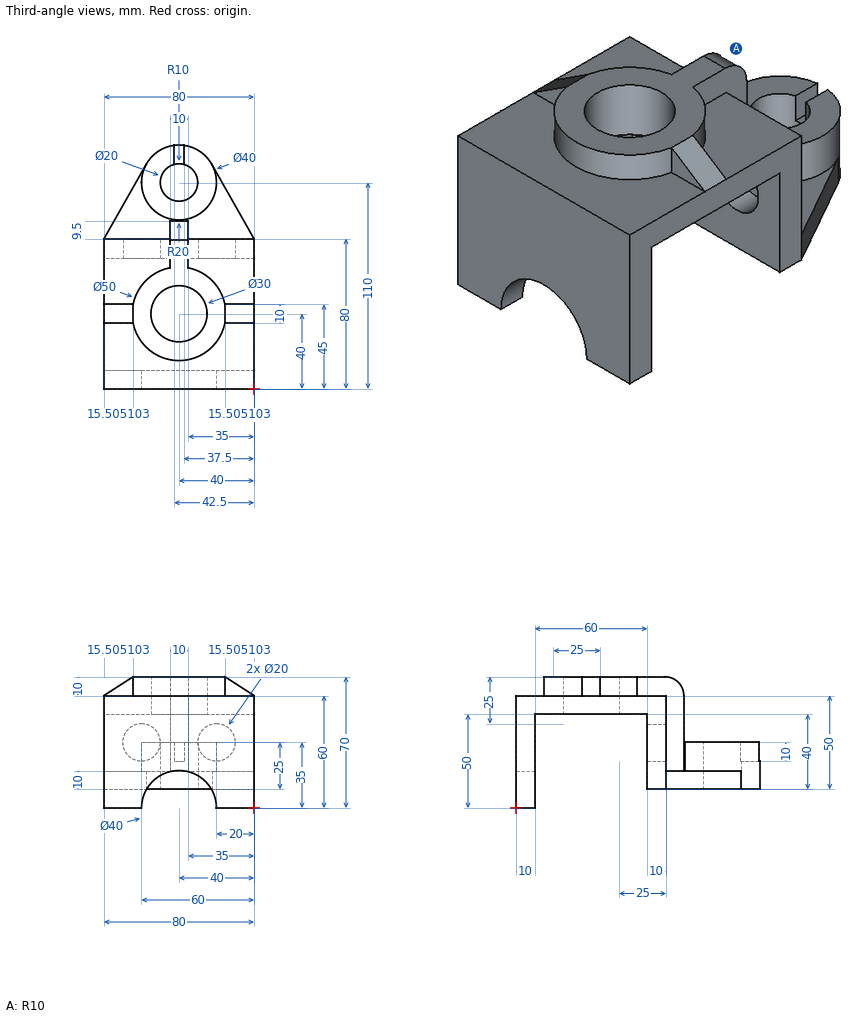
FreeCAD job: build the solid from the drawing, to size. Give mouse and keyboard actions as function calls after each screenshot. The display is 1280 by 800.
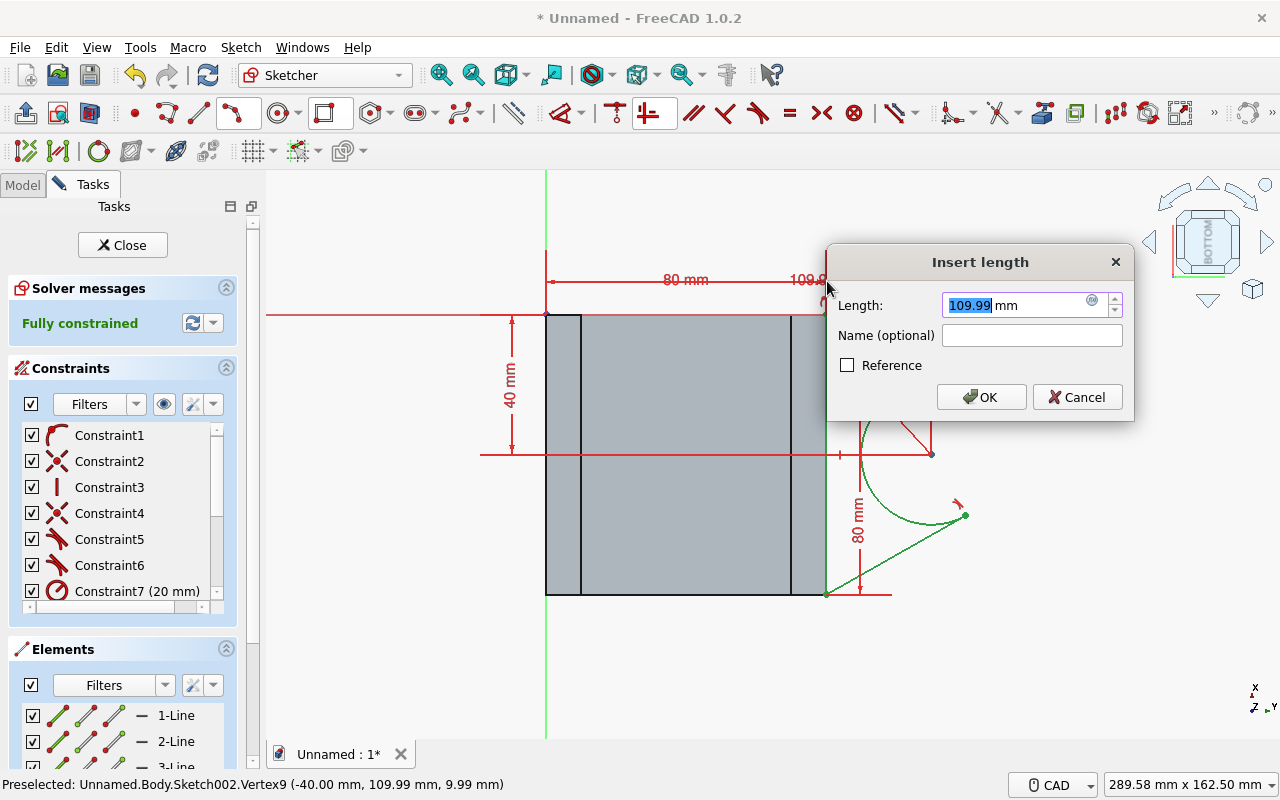
text(110)
key(Return)
key(Escape)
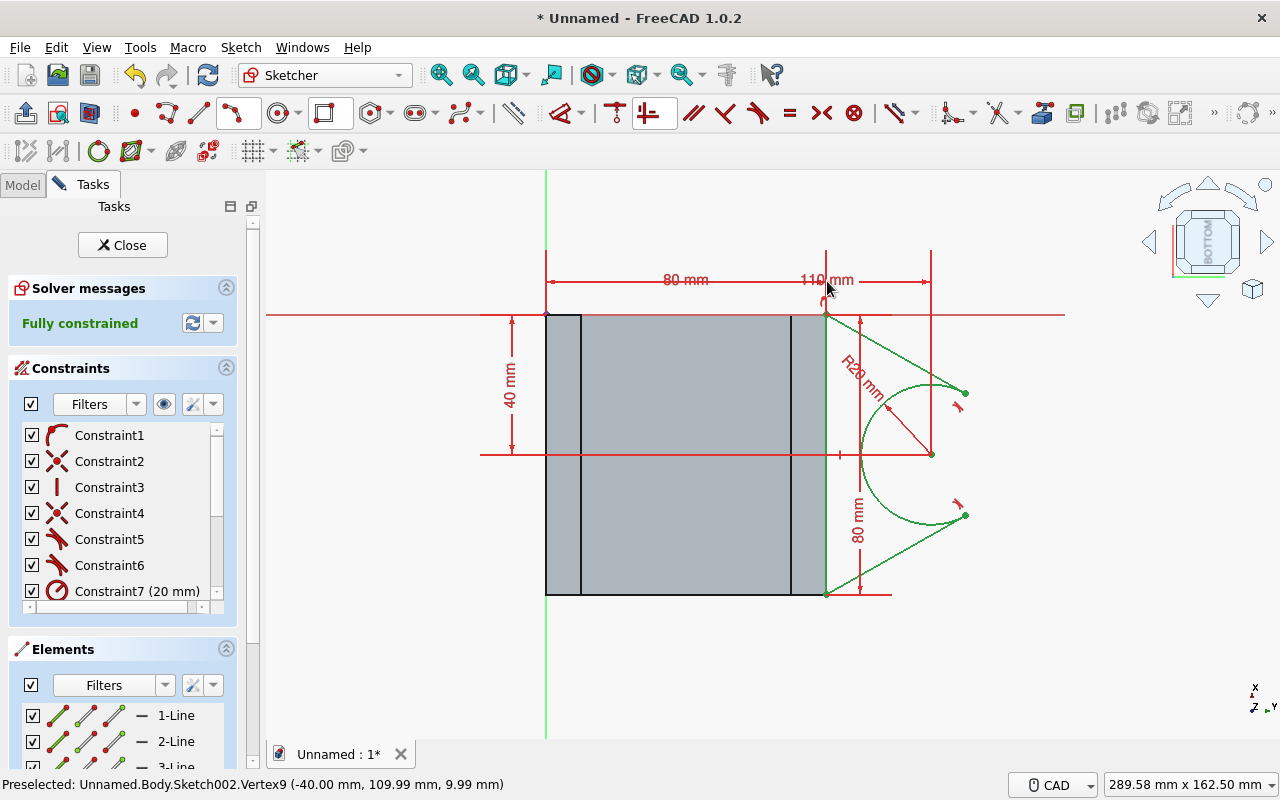
click(123, 245)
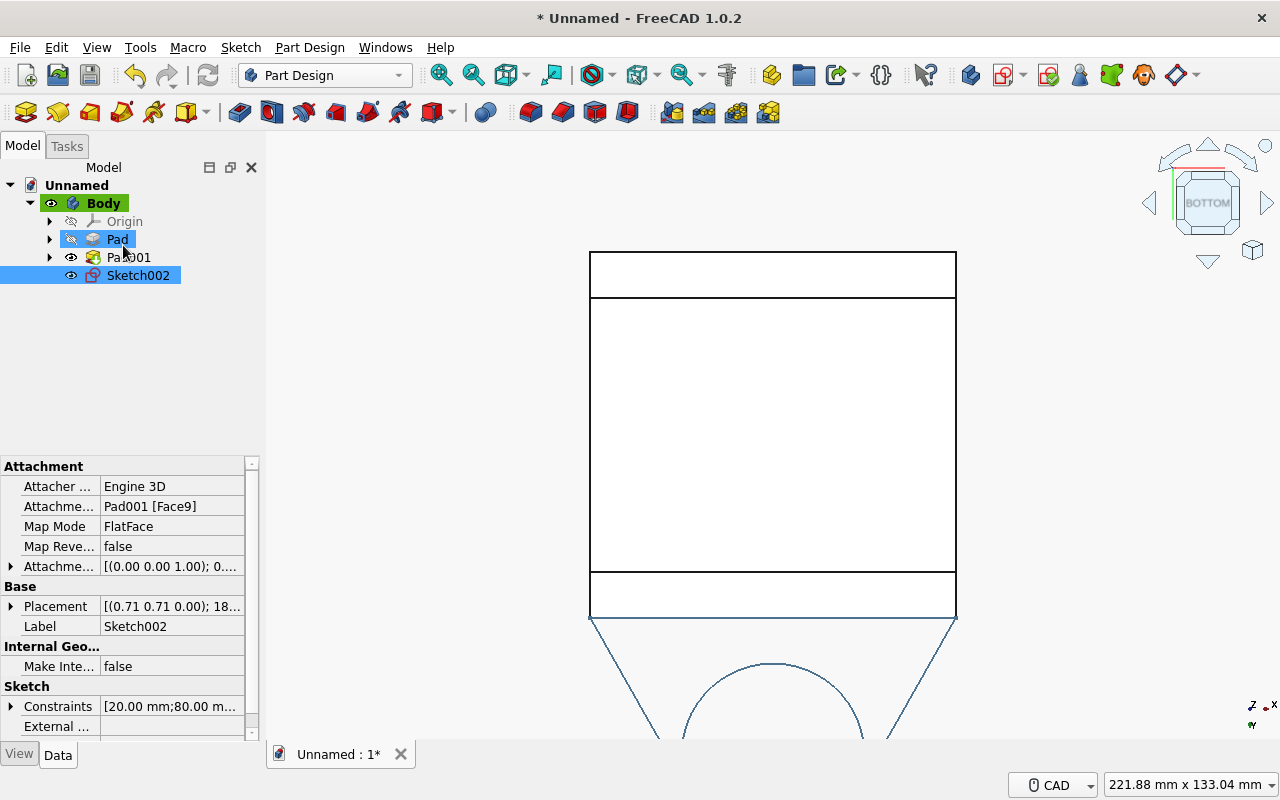
click(26, 112)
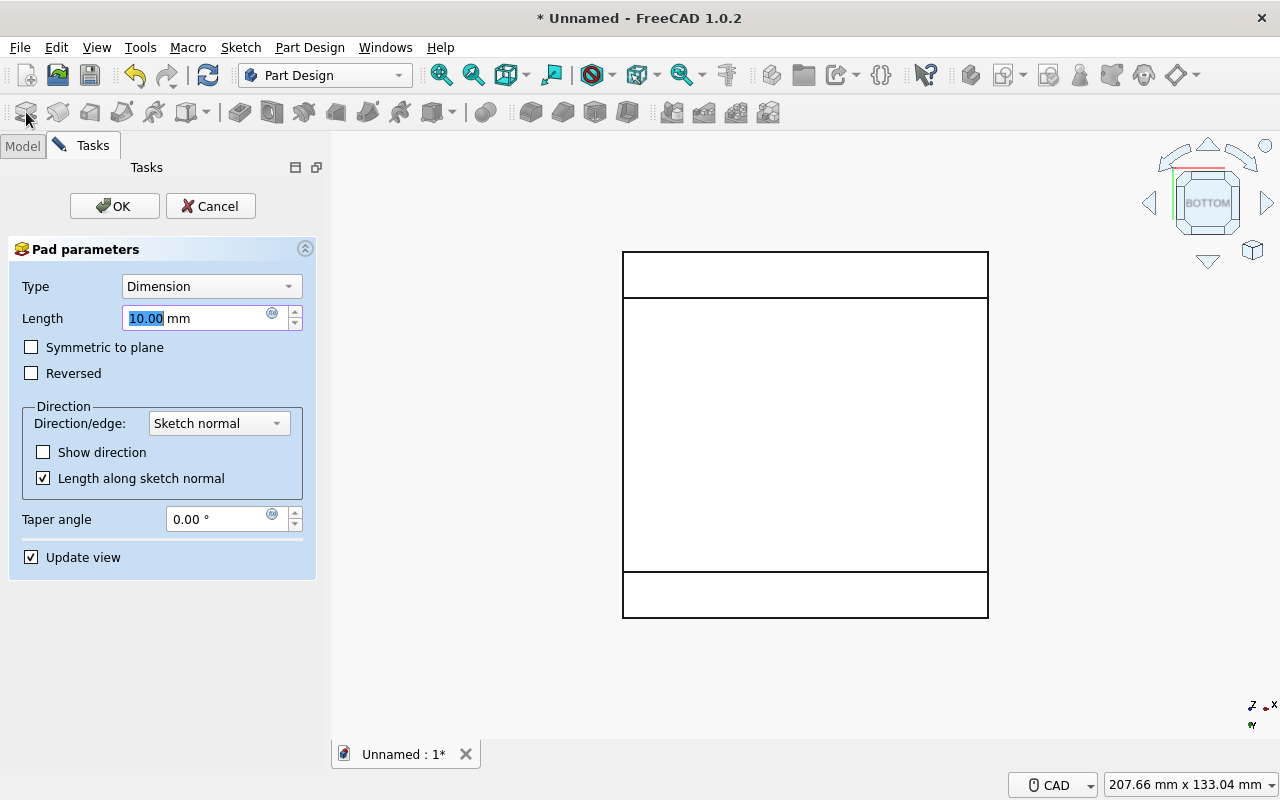
text(10)
key(Tab)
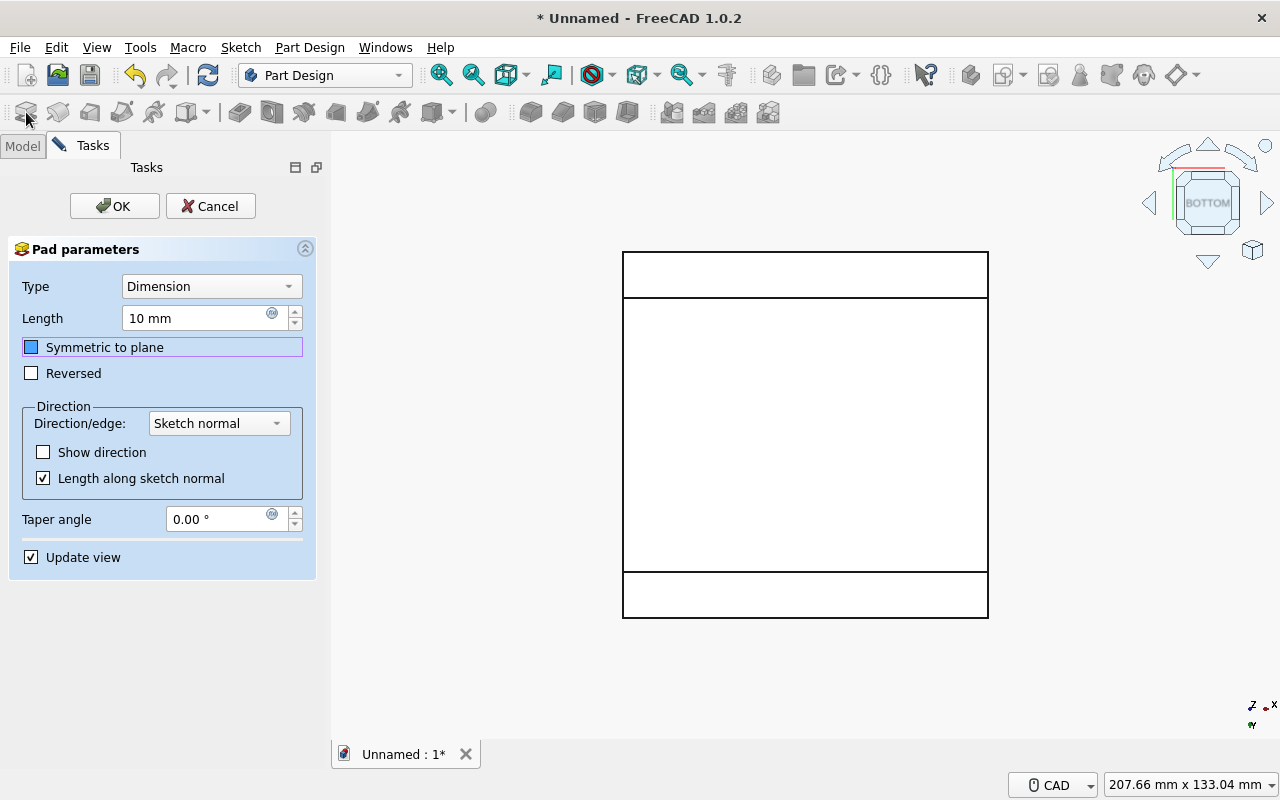
click(30, 373)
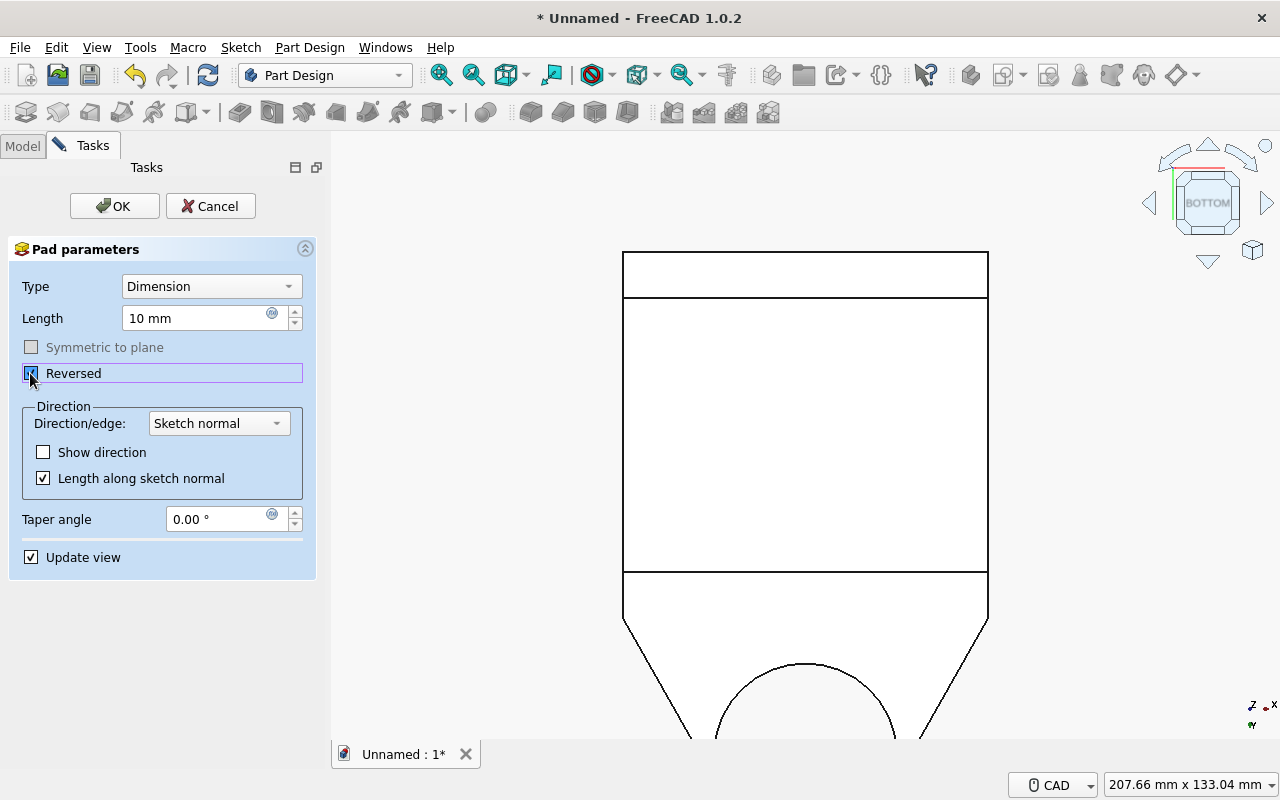
click(115, 206)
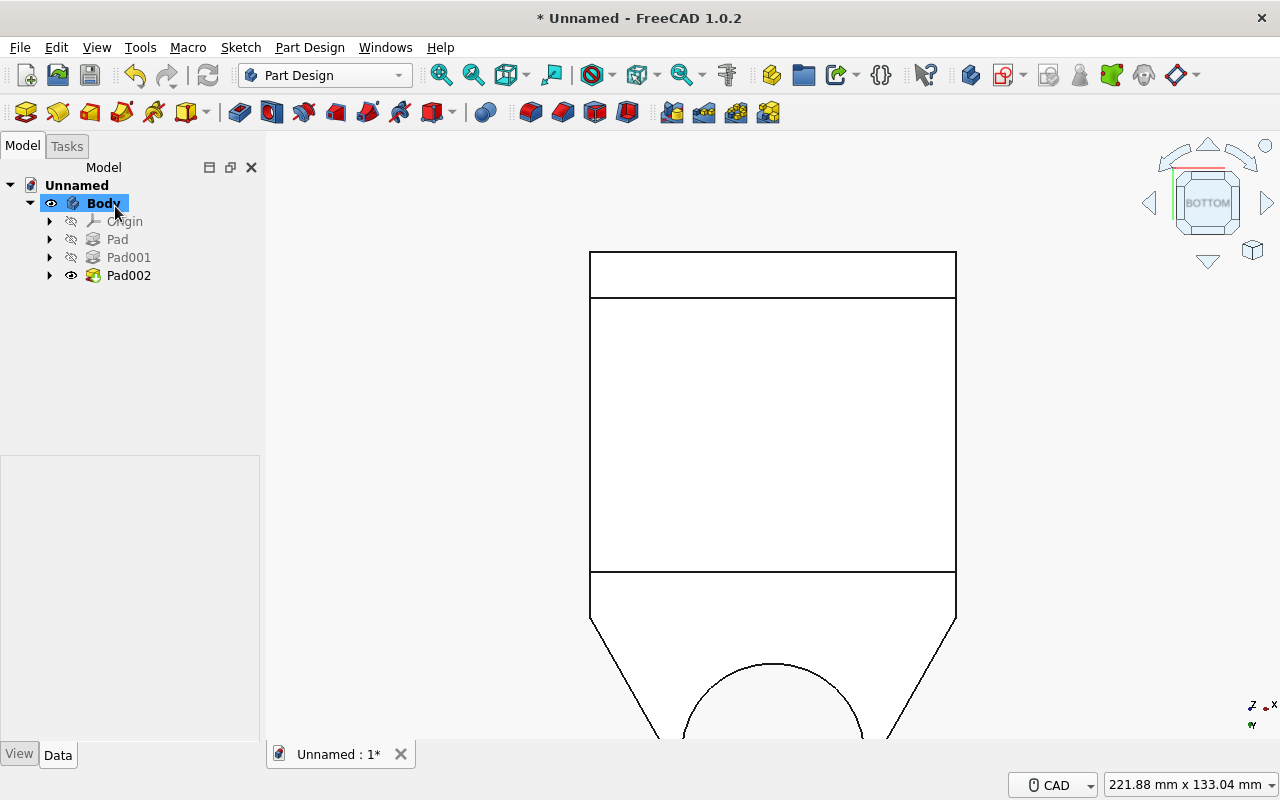
click(442, 76)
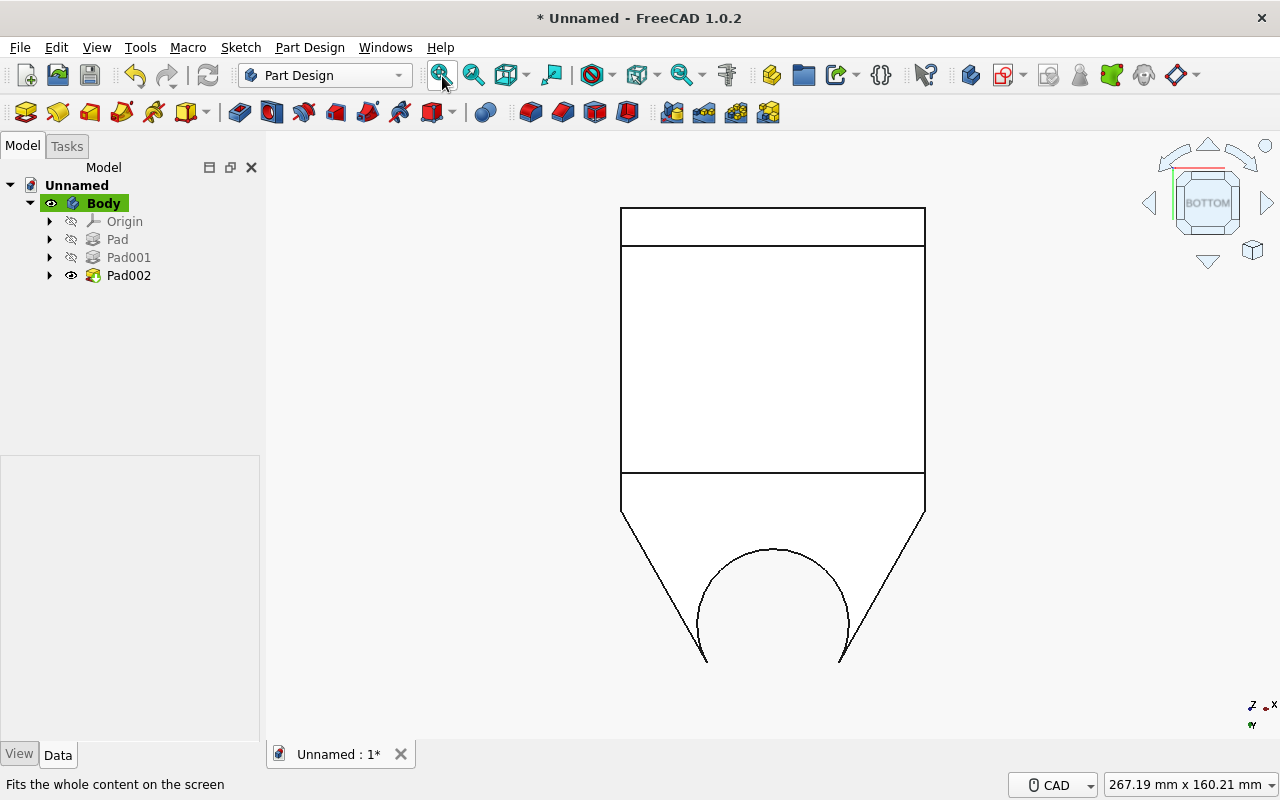
click(860, 540)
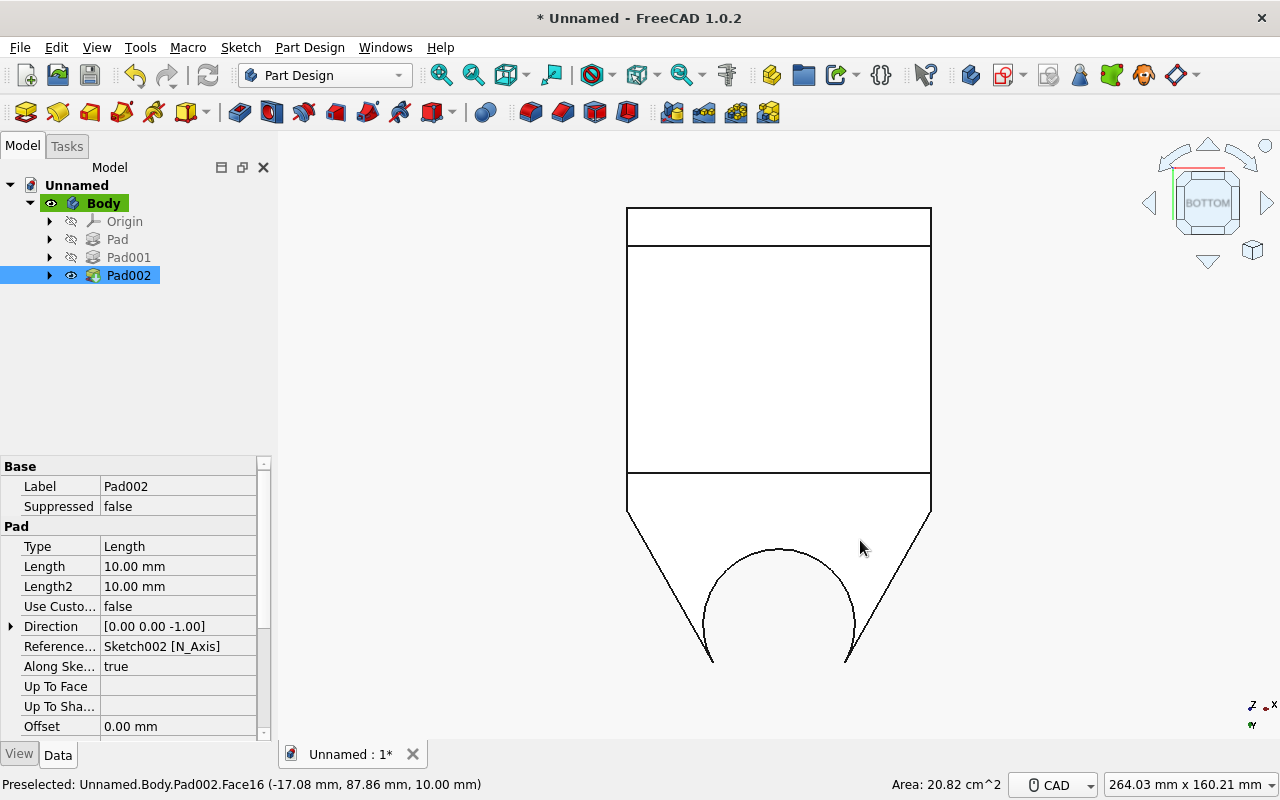
click(1004, 76)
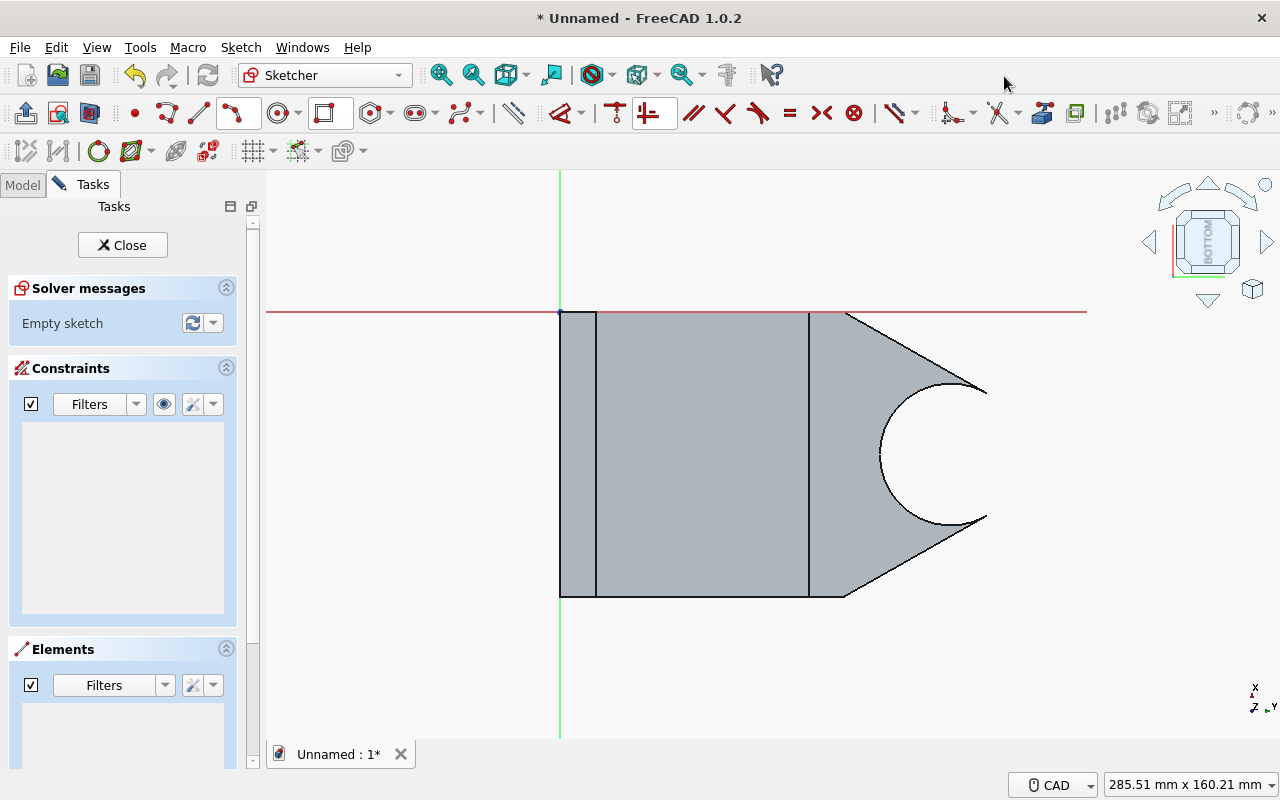
scroll(1094, 454, up, 5)